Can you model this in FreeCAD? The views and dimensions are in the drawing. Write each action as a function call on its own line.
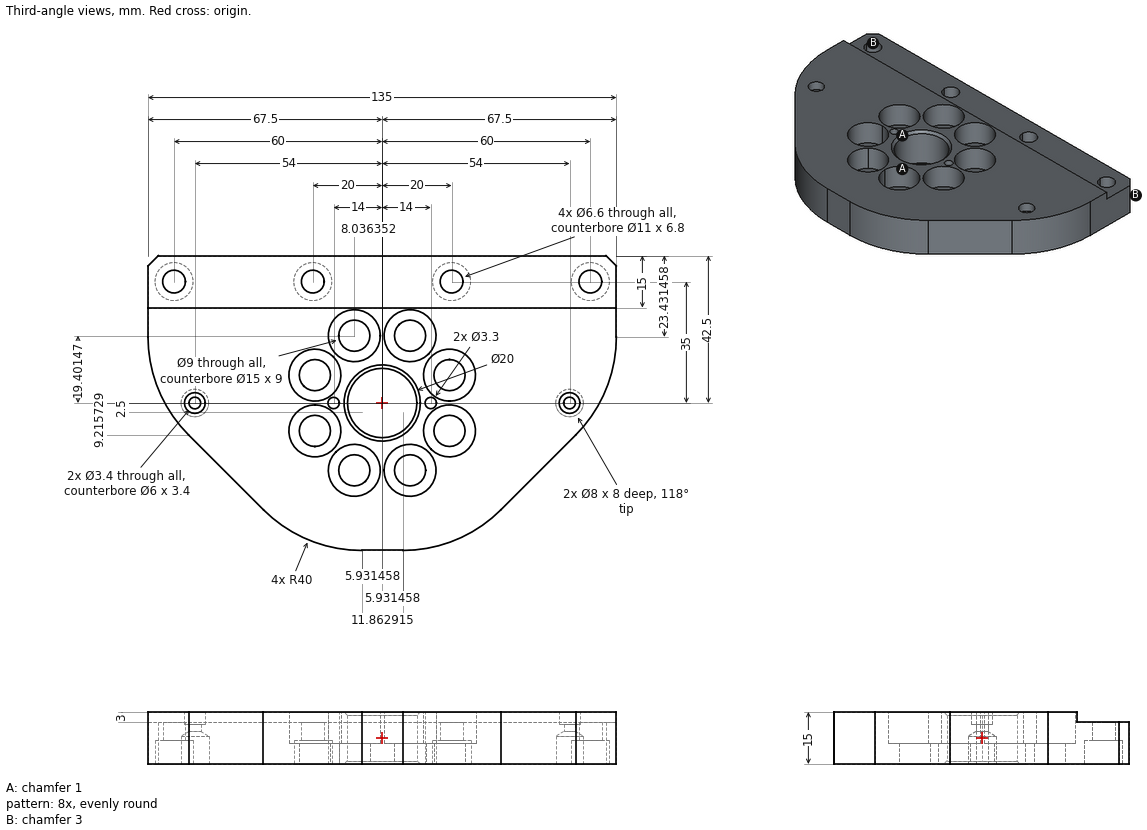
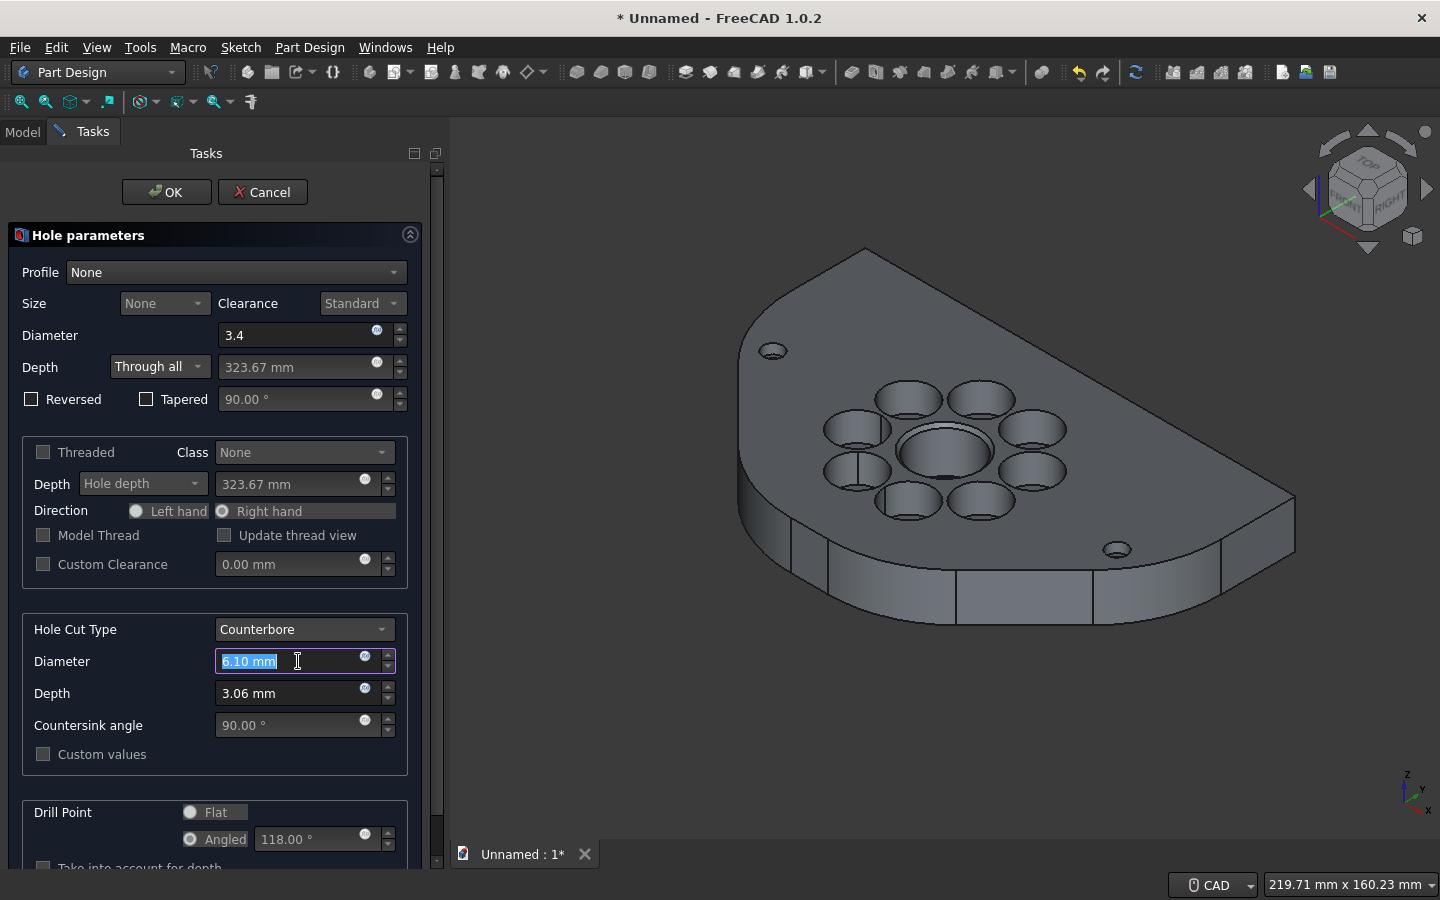
text(6)
key(Tab)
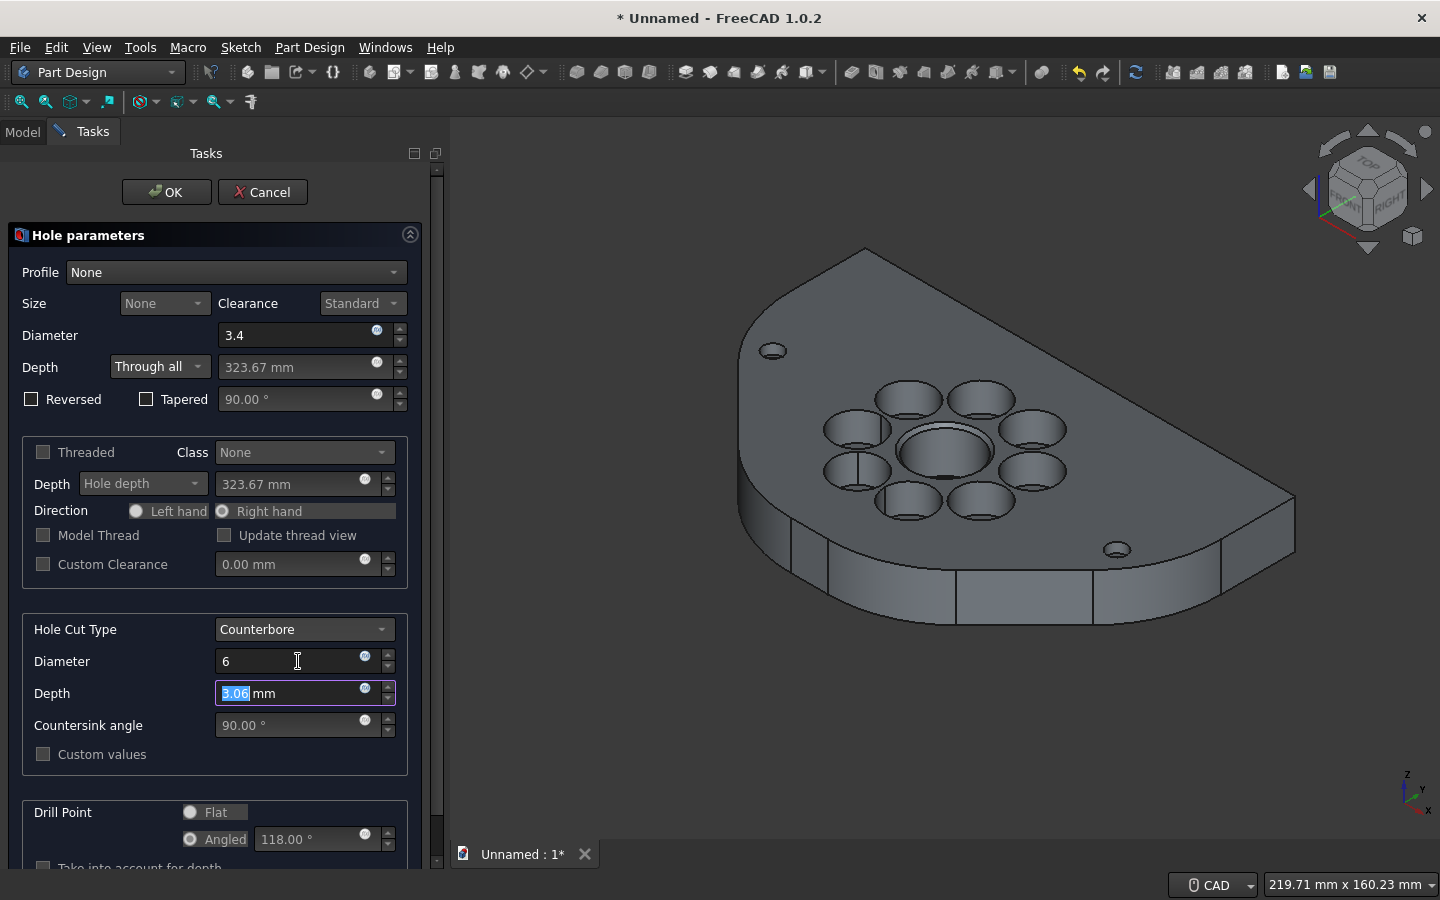
text(3.4)
key(Tab)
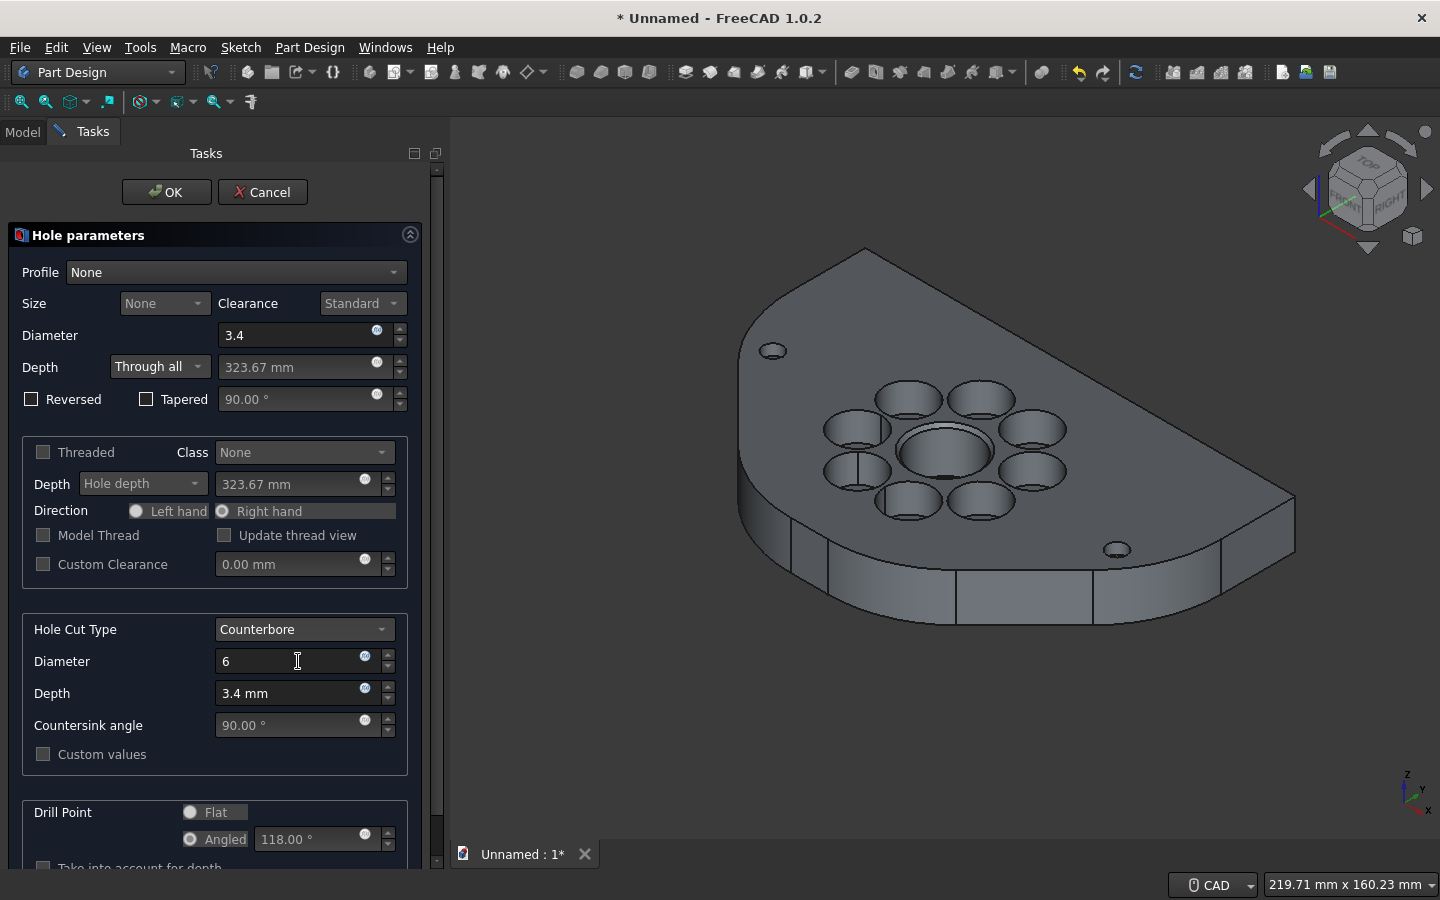
click(167, 192)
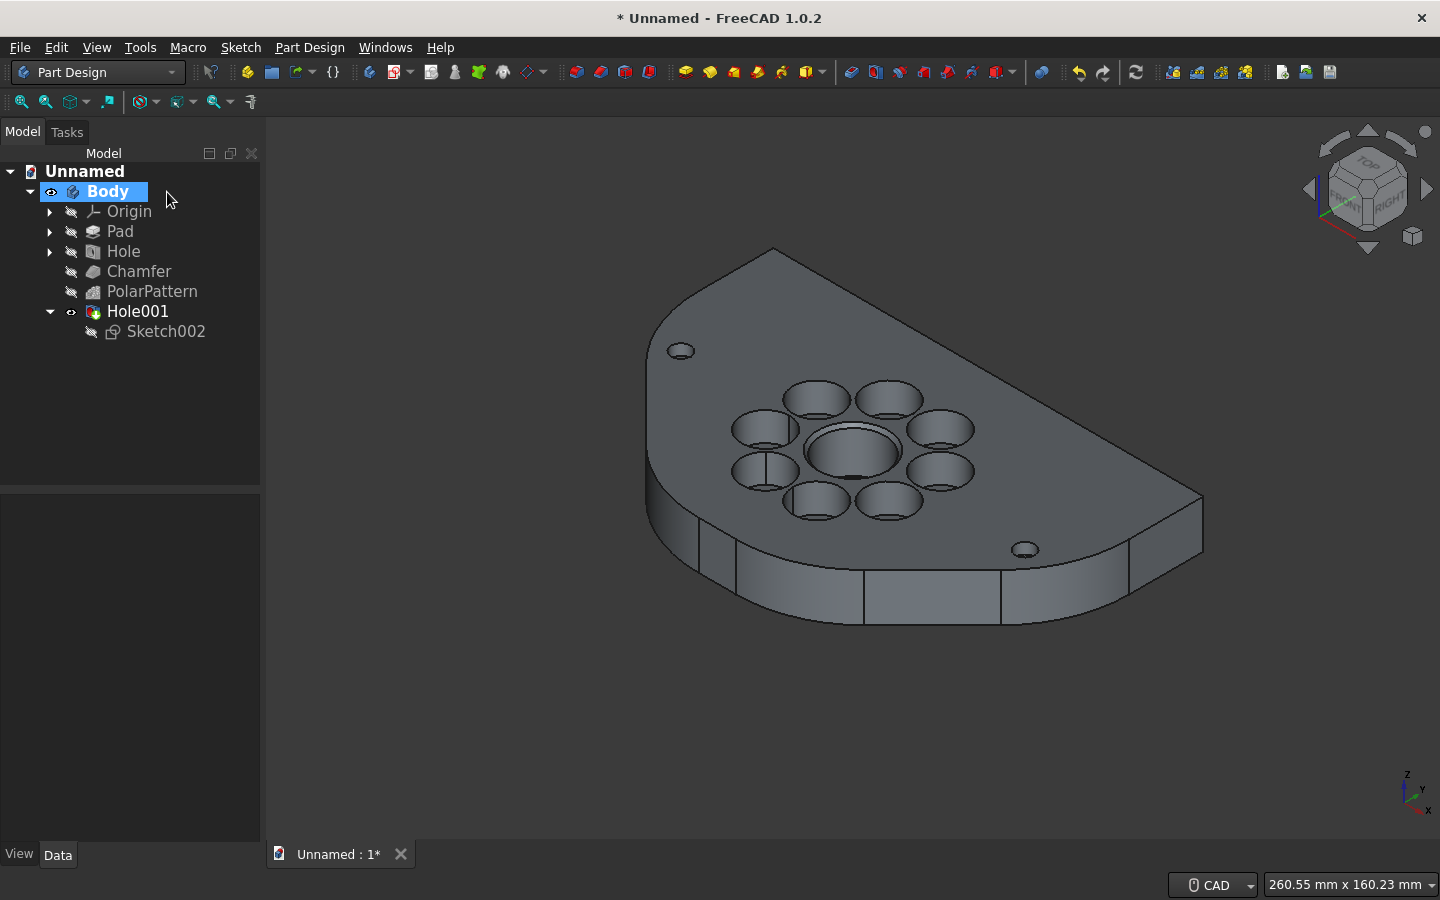
key(5)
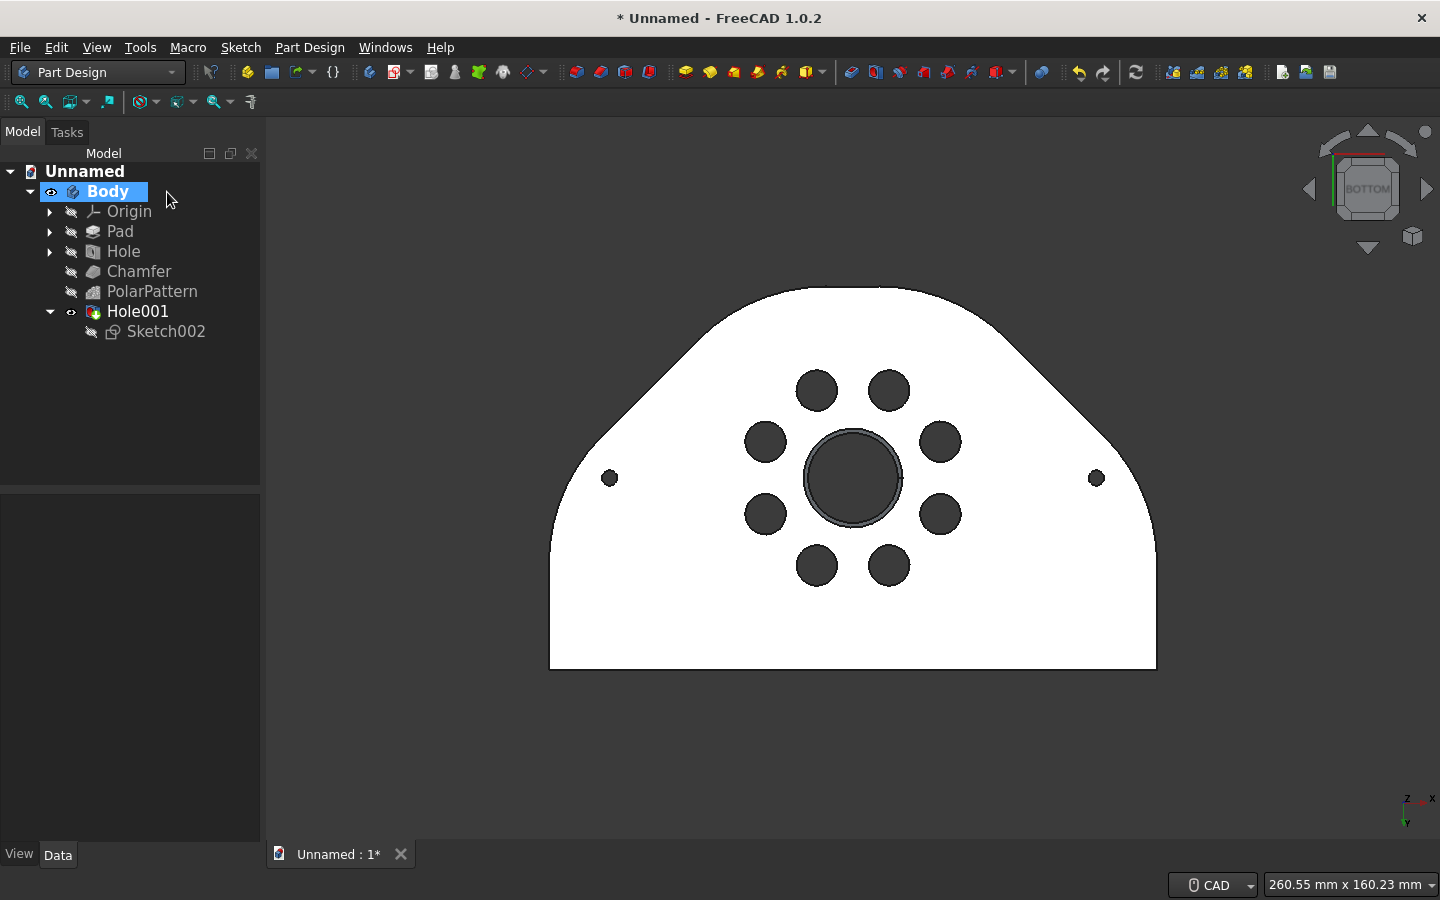
click(1027, 586)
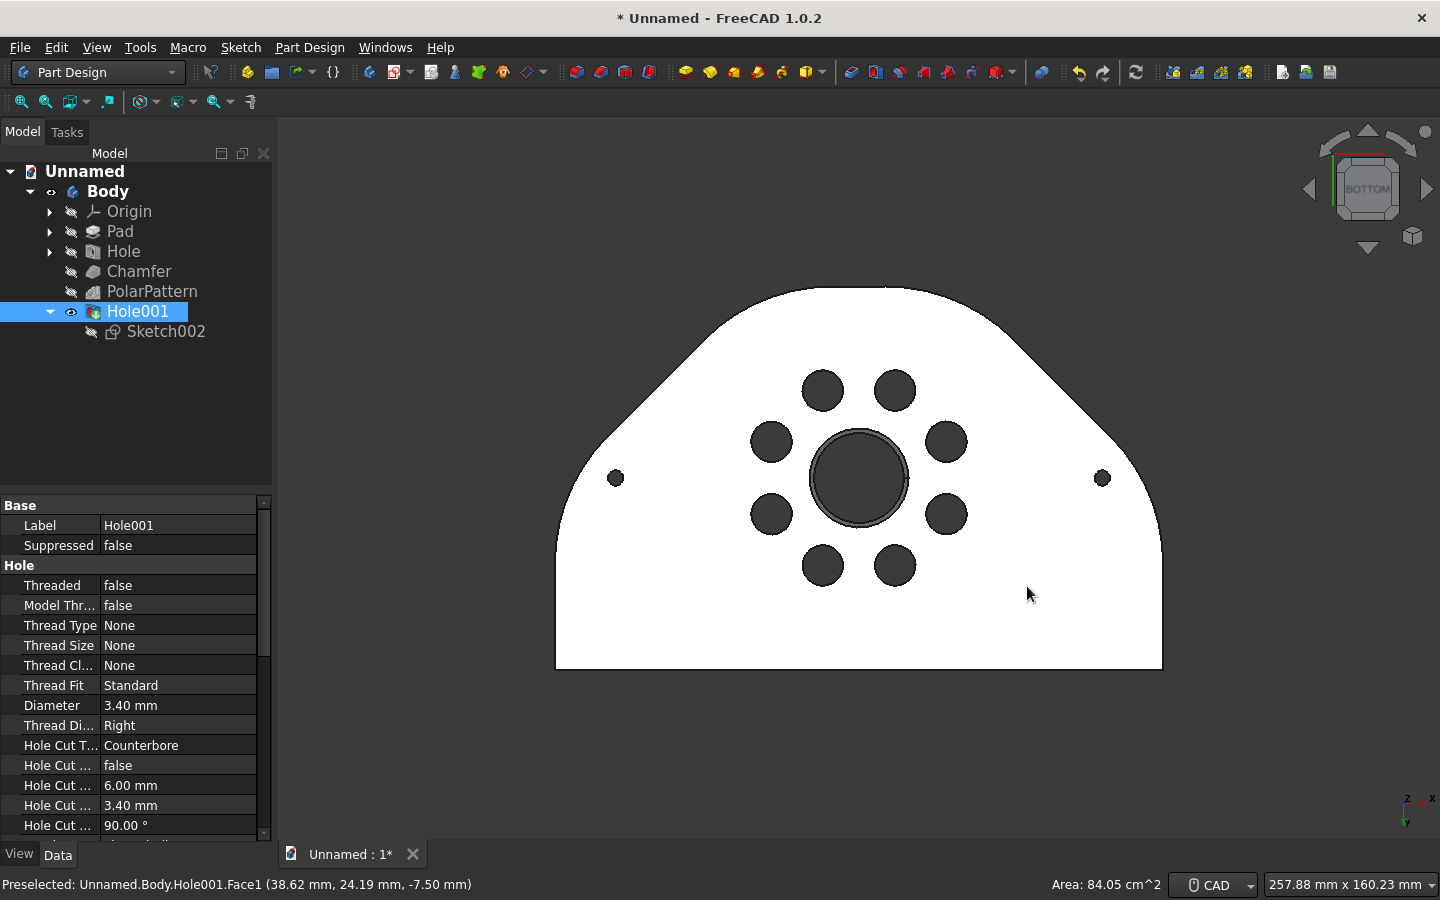
click(394, 72)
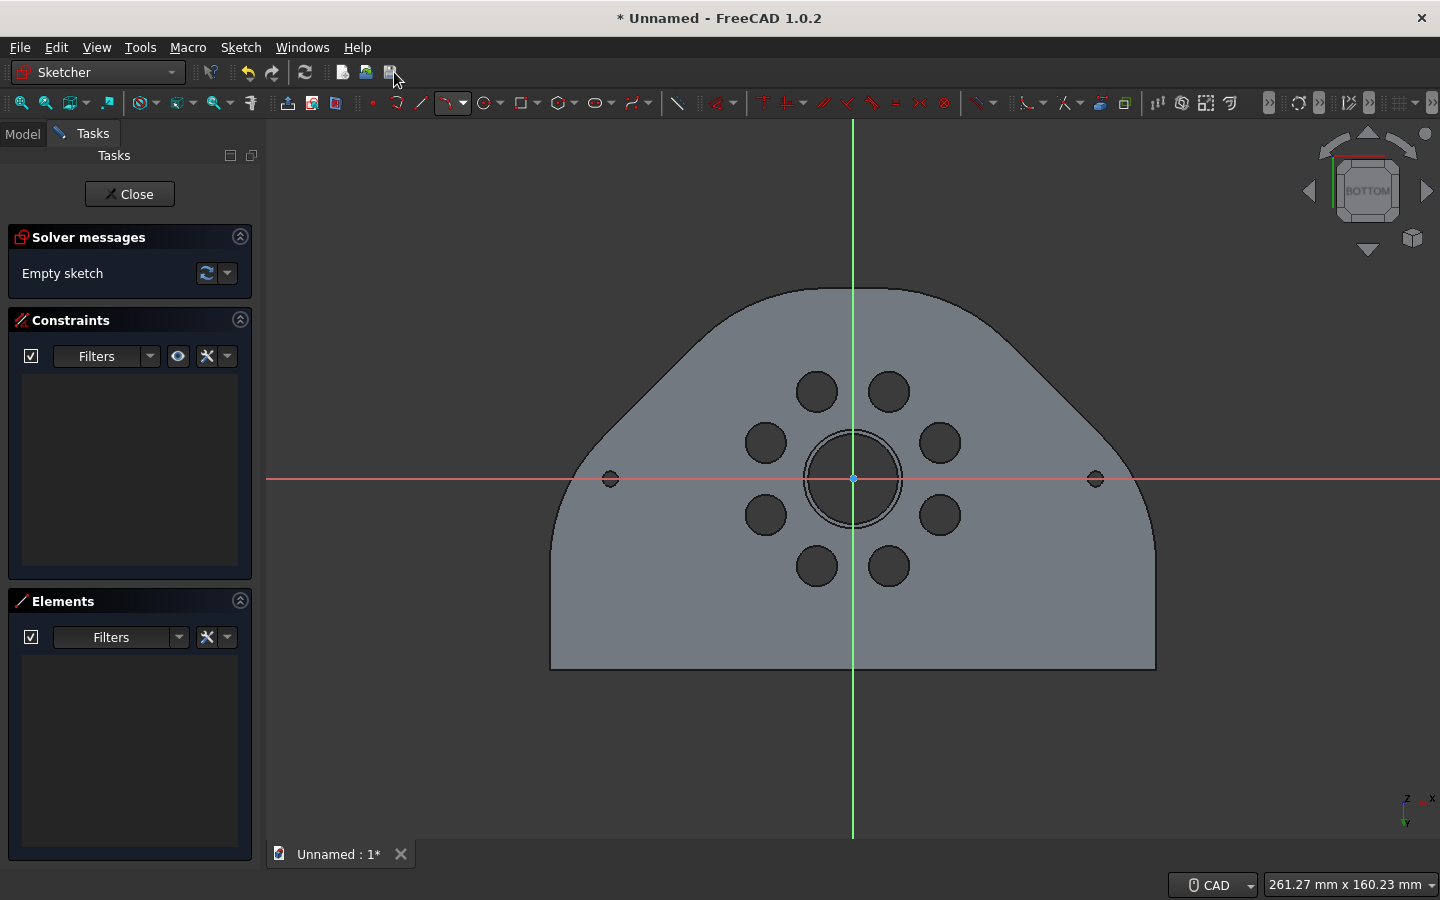
key(g)
key(c)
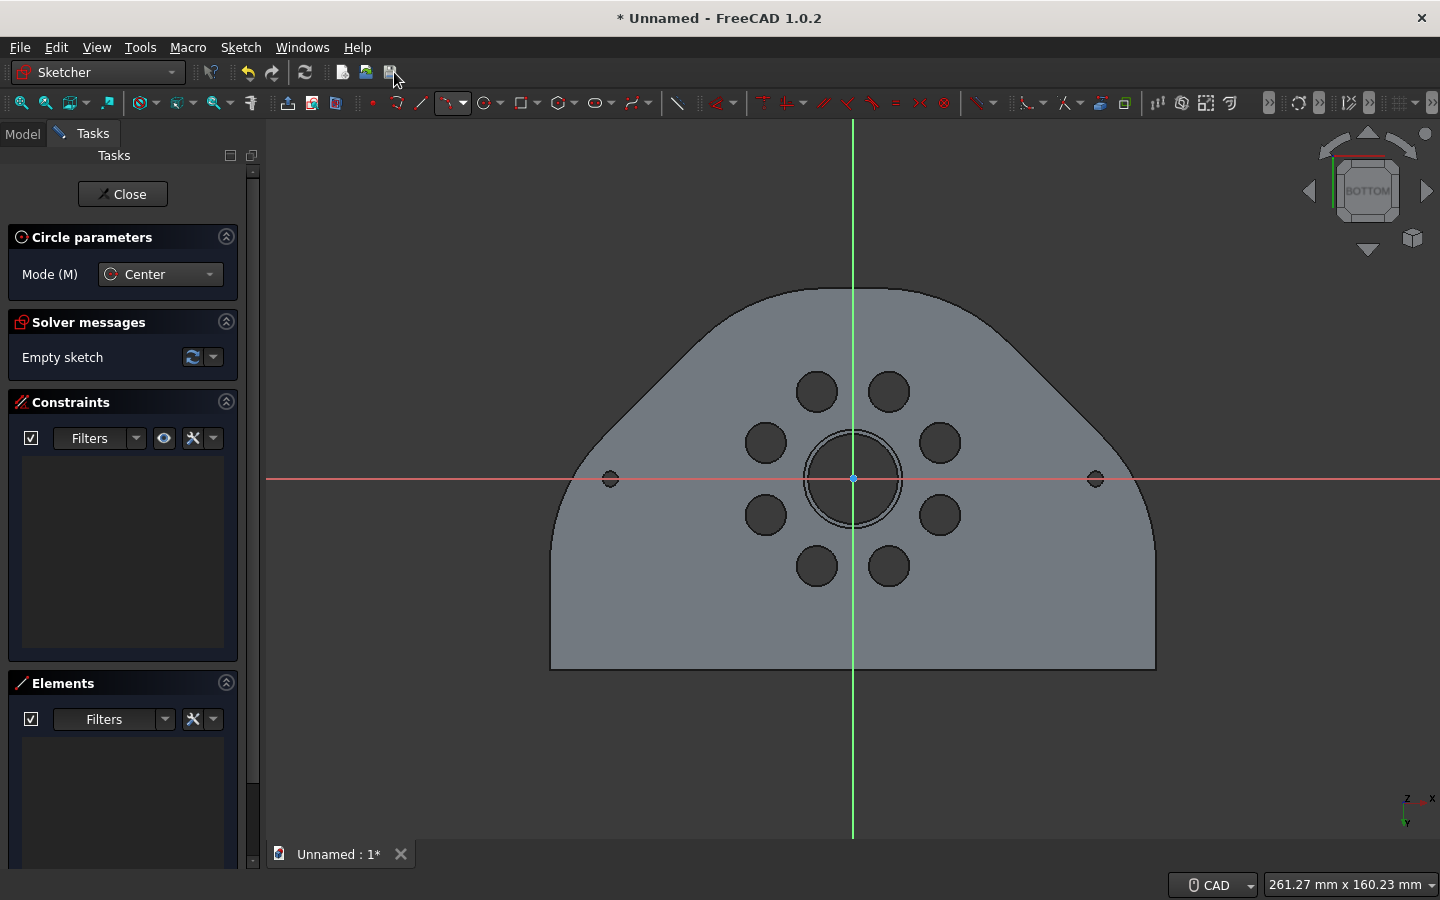
scroll(1096, 479, up, 2)